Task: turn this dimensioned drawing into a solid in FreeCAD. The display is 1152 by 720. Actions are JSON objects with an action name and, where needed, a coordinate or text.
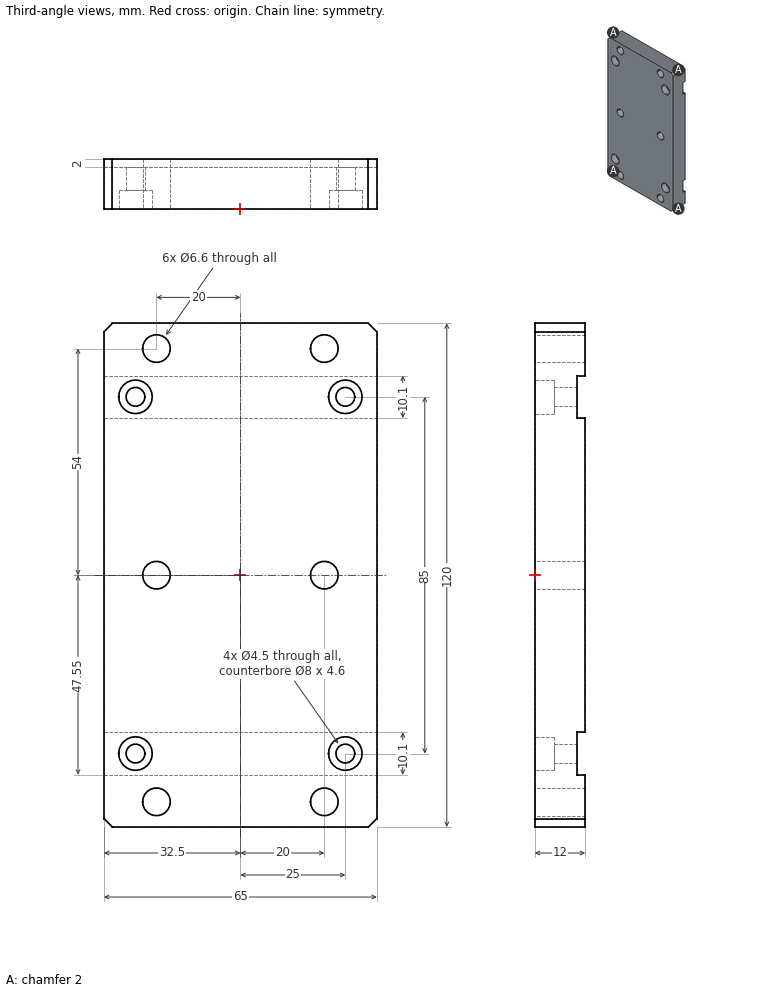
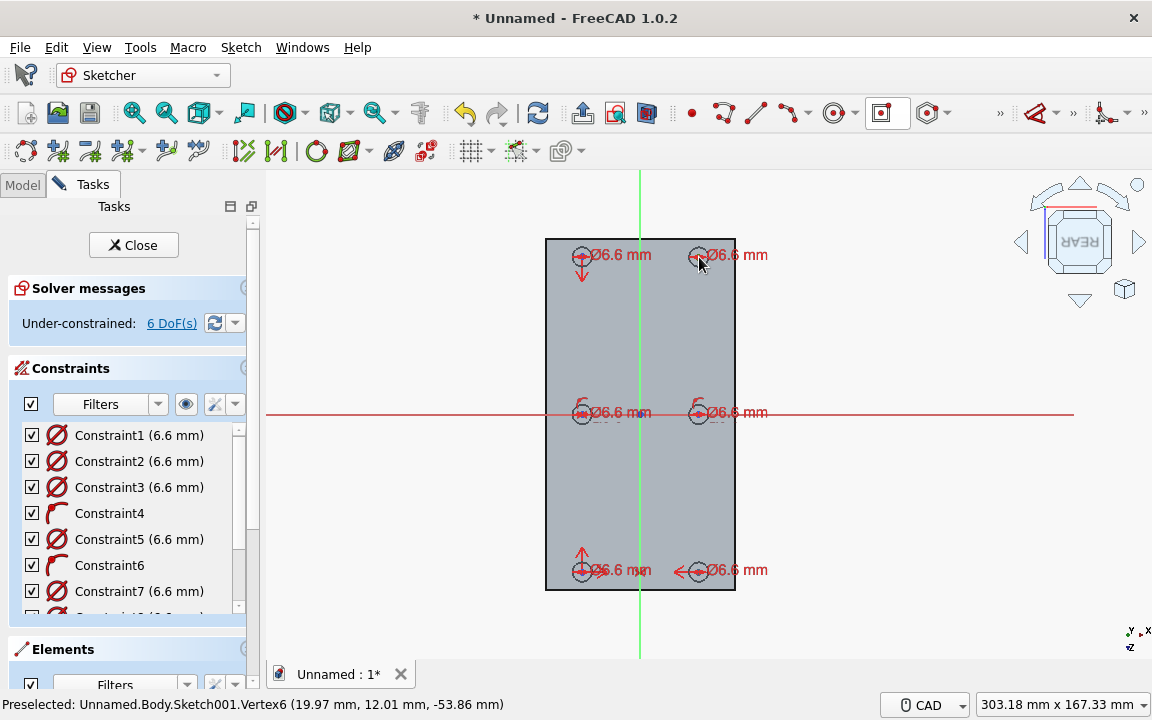
{"action": "left_click", "coordinate": [344, 414]}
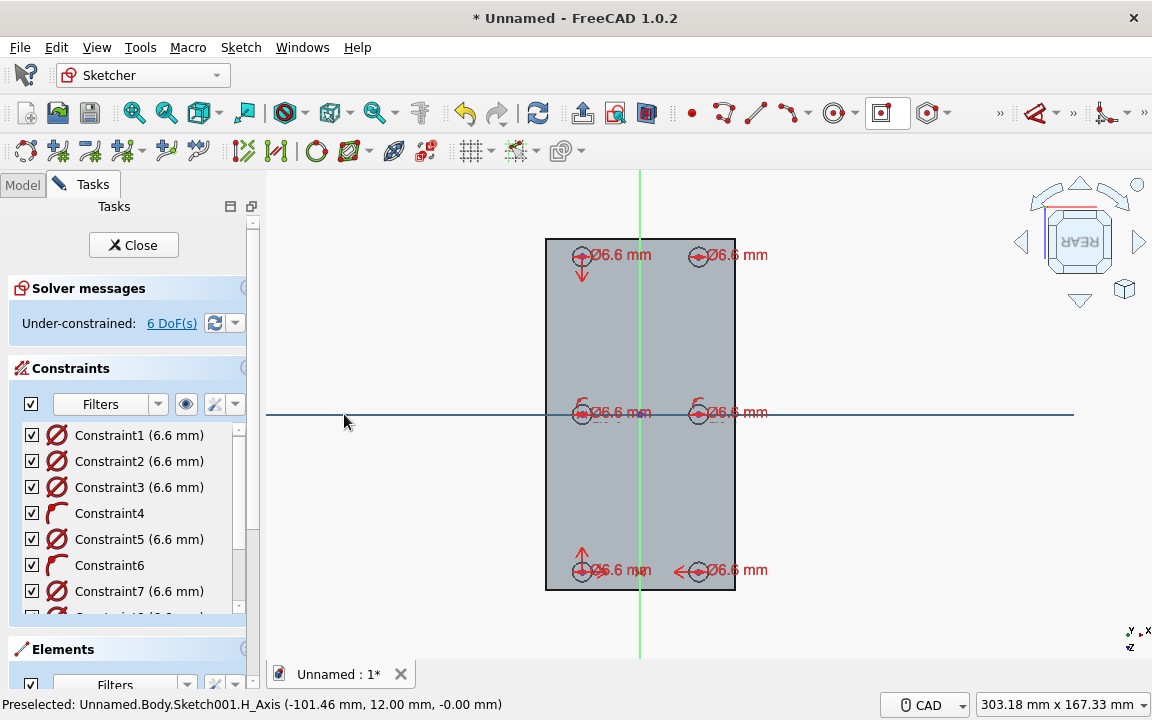
{"action": "key", "text": "s"}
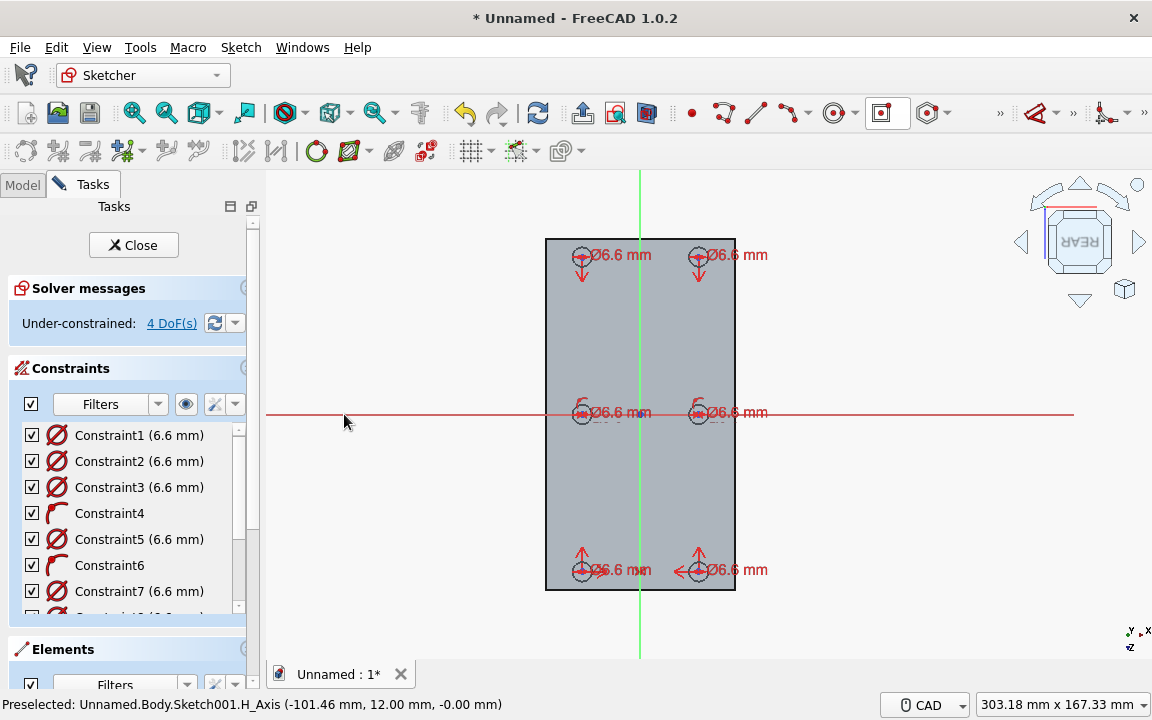
{"action": "key", "text": "d"}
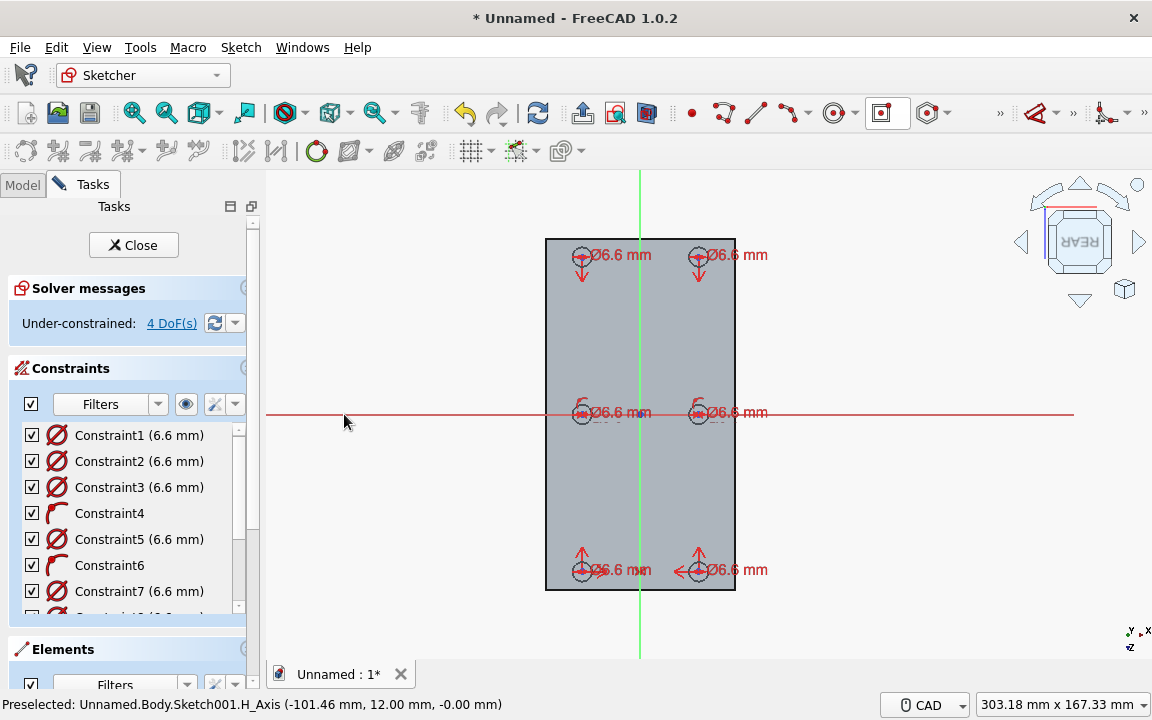
{"action": "left_click", "coordinate": [582, 572]}
{"action": "left_click", "coordinate": [611, 606]}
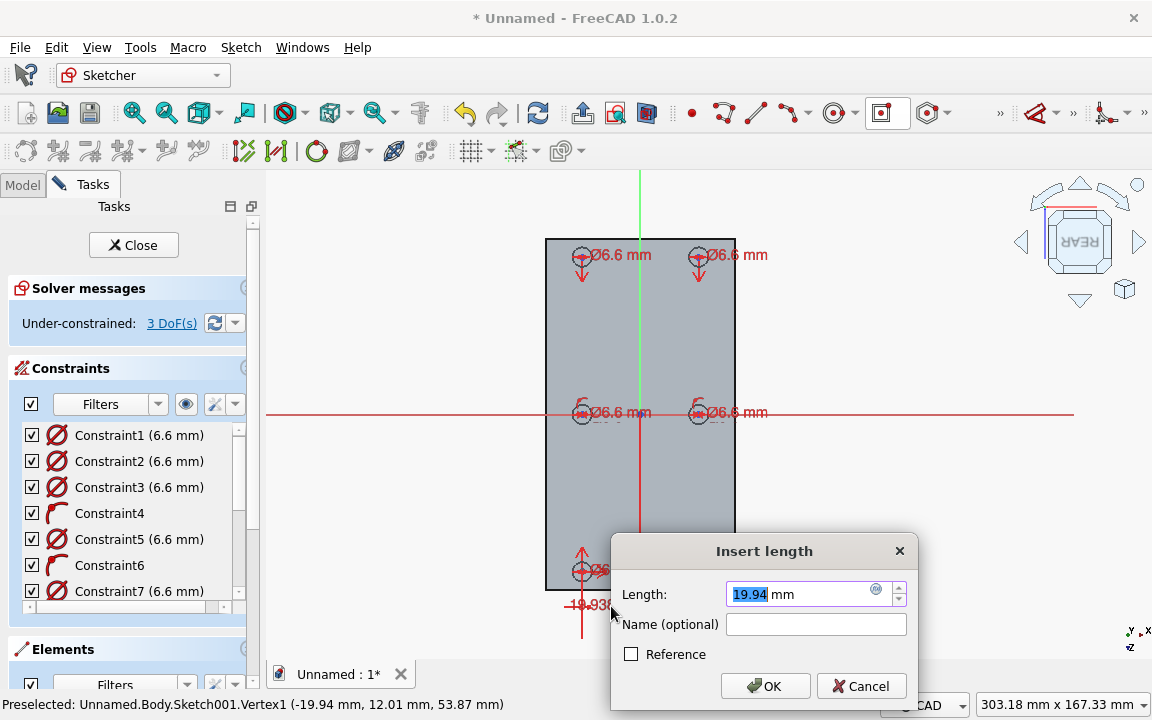
{"action": "type", "text": "20"}
{"action": "key", "text": "Return"}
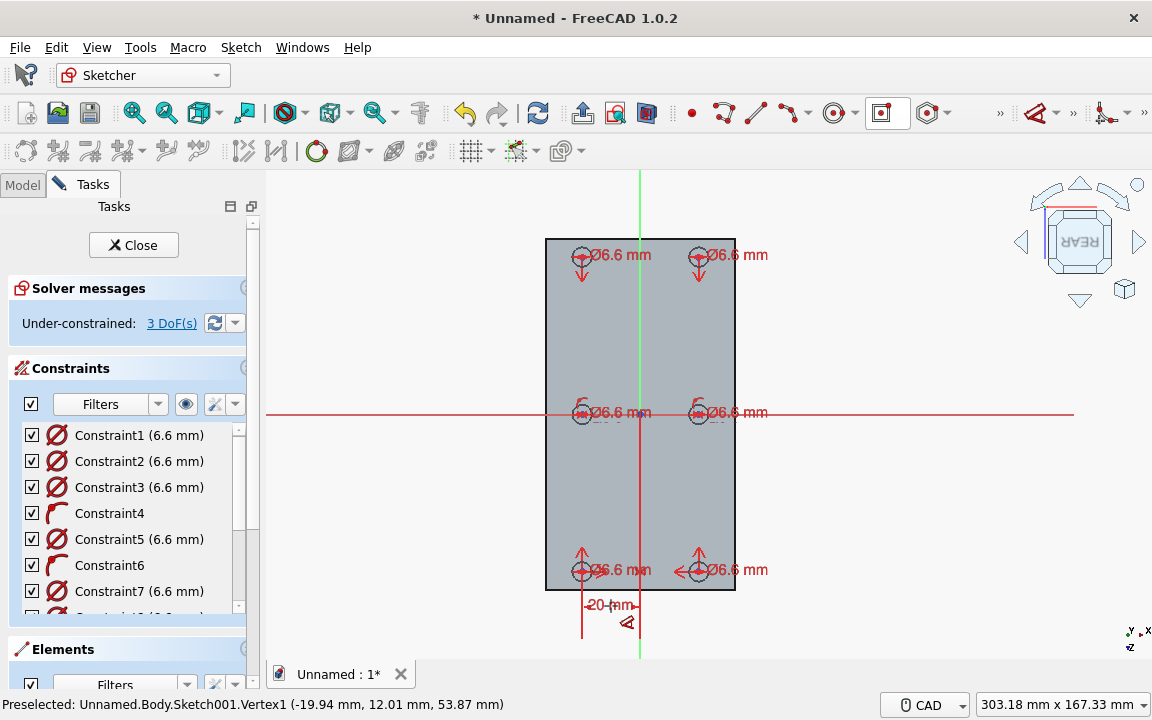
{"action": "left_click", "coordinate": [582, 572]}
{"action": "left_click", "coordinate": [548, 493]}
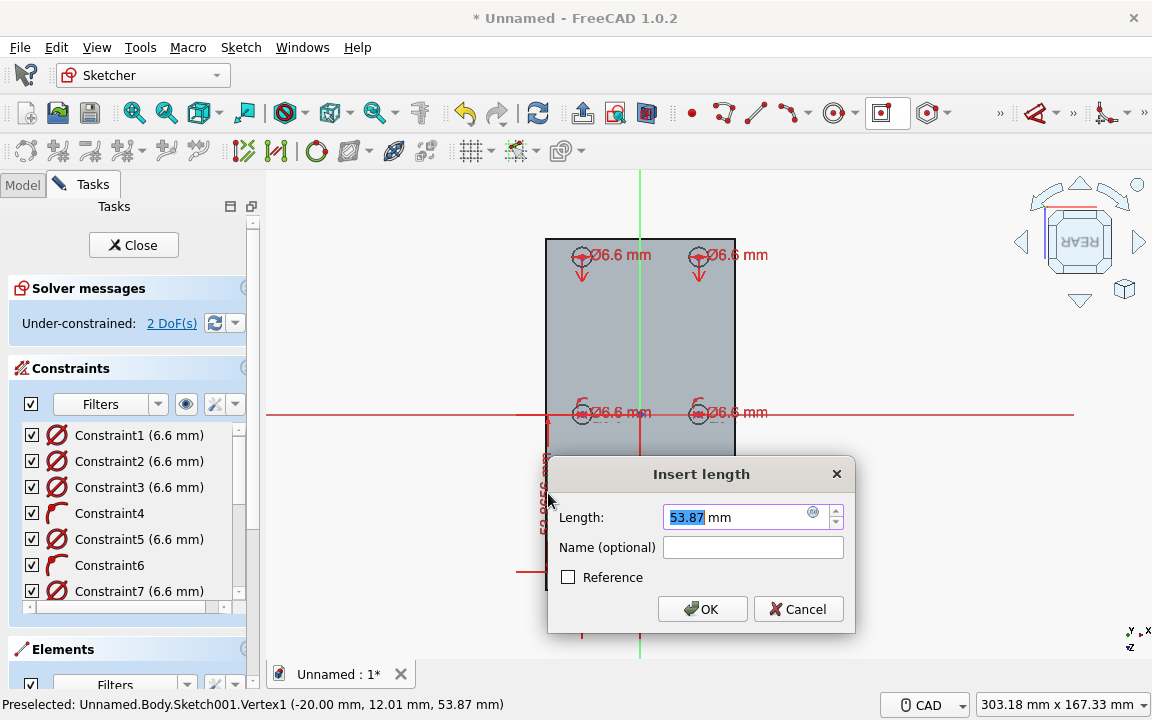
{"action": "type", "text": "54"}
{"action": "key", "text": "Return"}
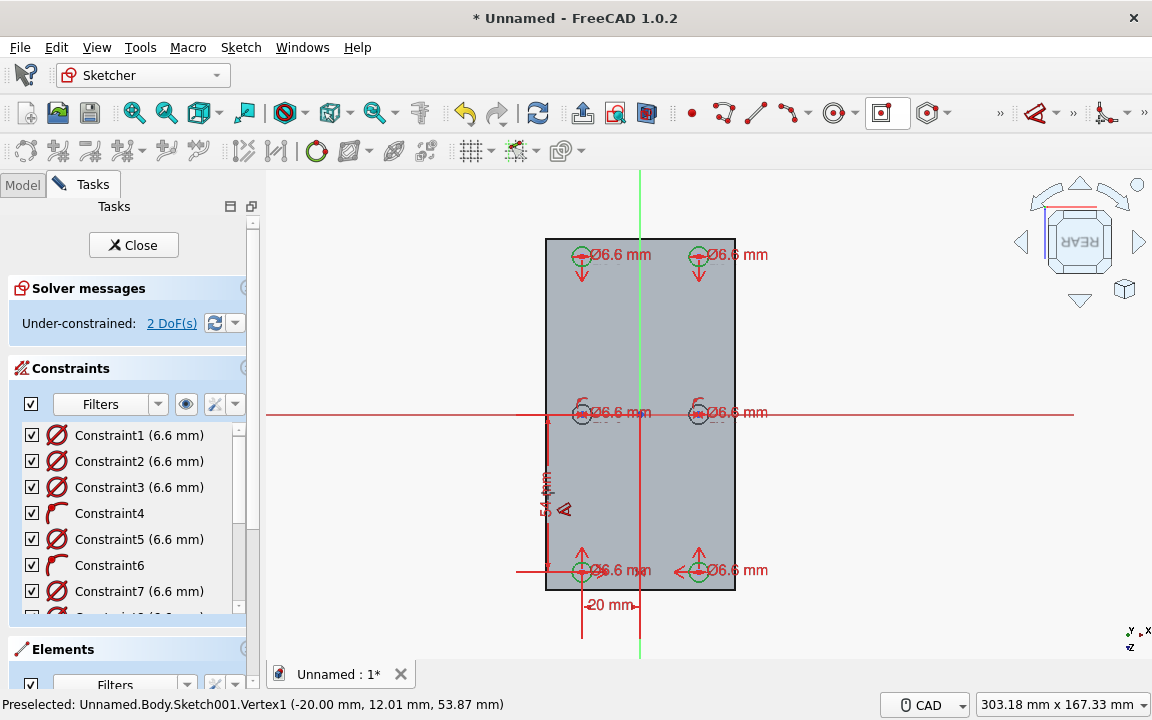
{"action": "left_click", "coordinate": [582, 414]}
{"action": "left_click", "coordinate": [611, 448]}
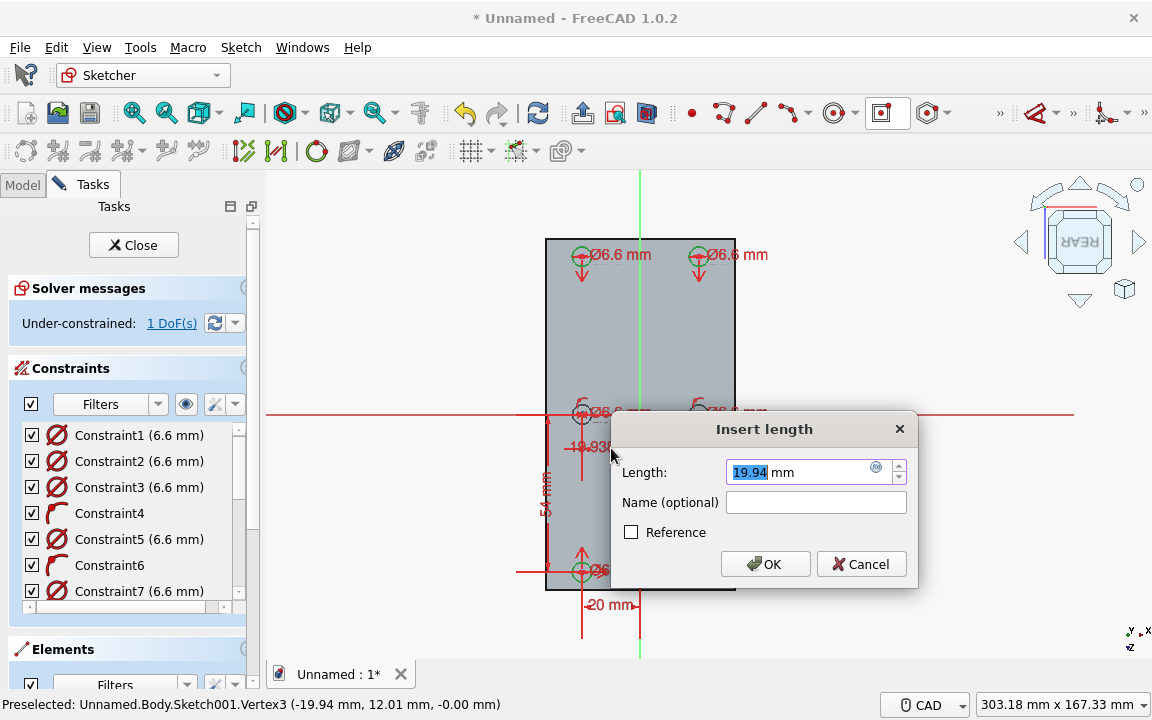
{"action": "type", "text": "20"}
{"action": "key", "text": "Return"}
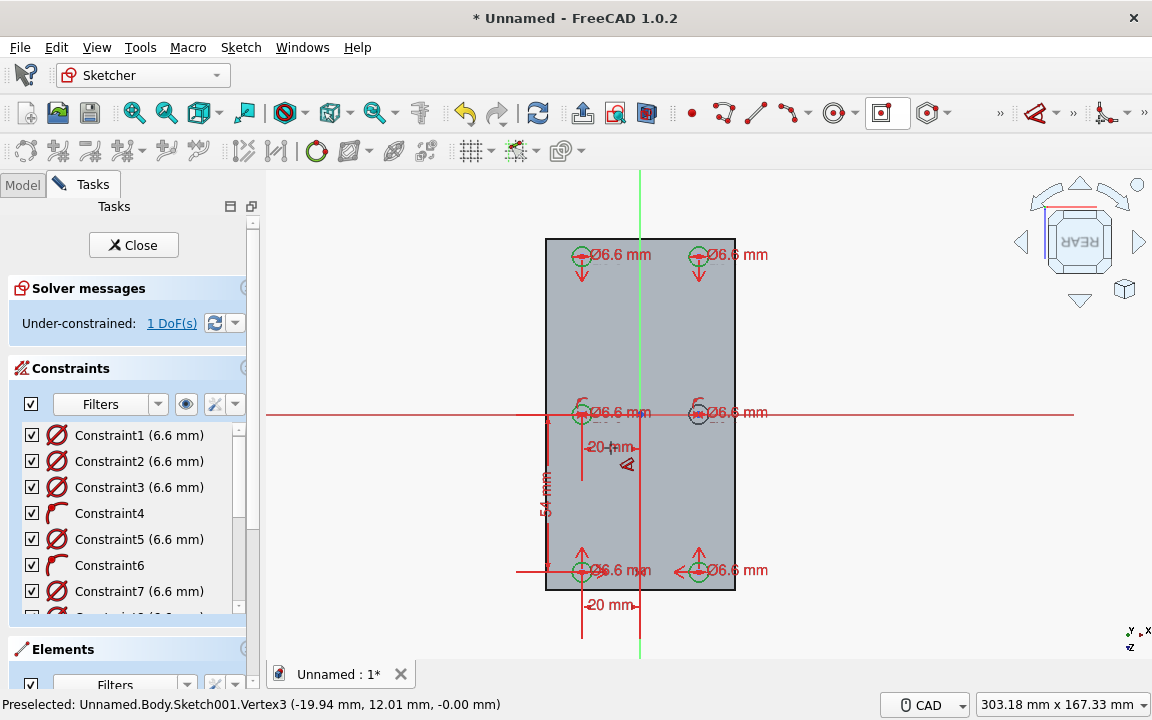
{"action": "left_click", "coordinate": [699, 414]}
{"action": "left_click", "coordinate": [683, 448]}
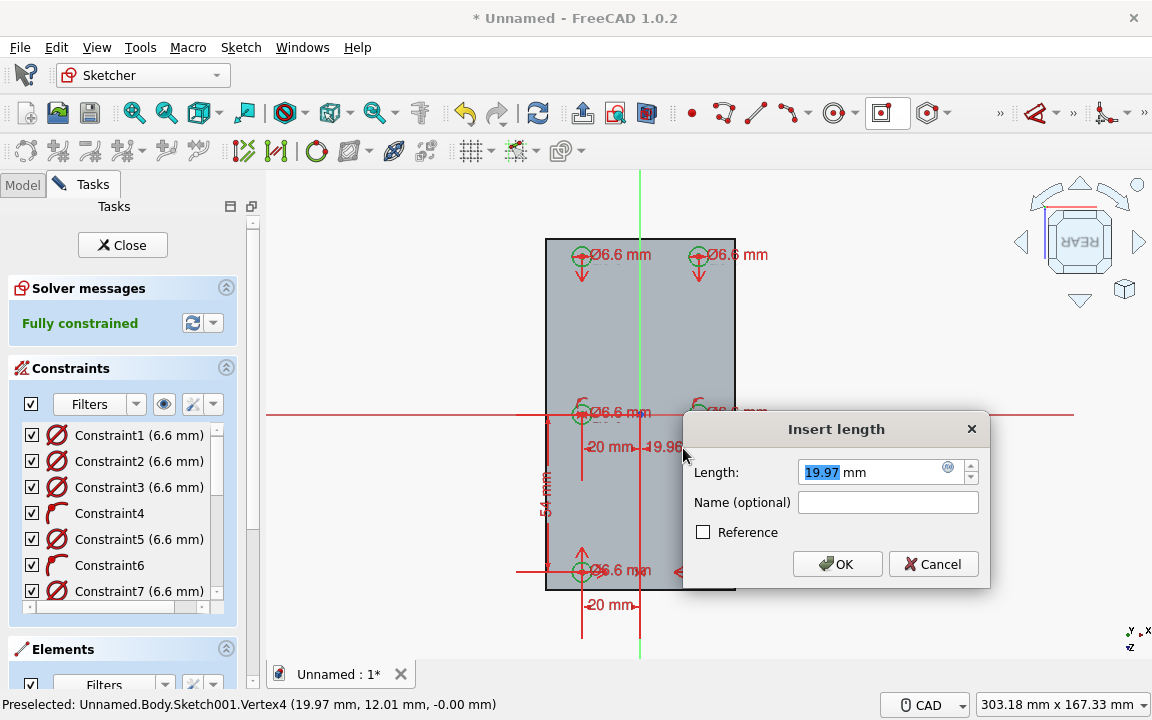
{"action": "type", "text": "20"}
{"action": "key", "text": "Return"}
{"action": "key", "text": "Escape"}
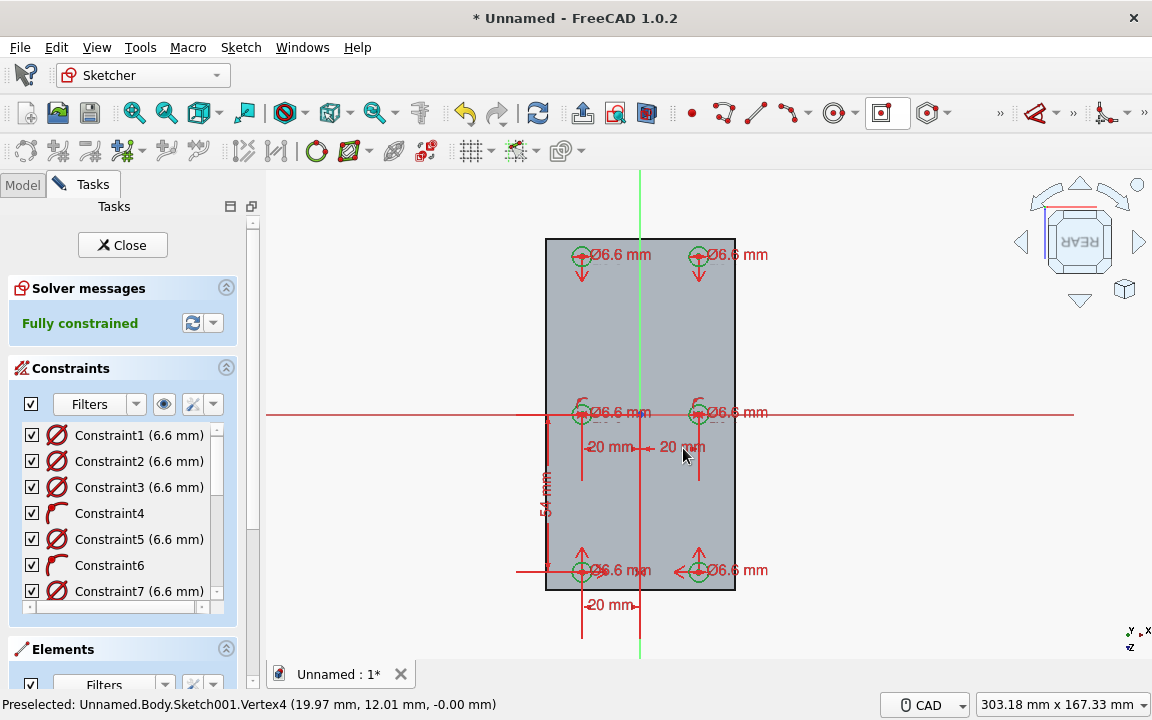
{"action": "left_click", "coordinate": [123, 245]}